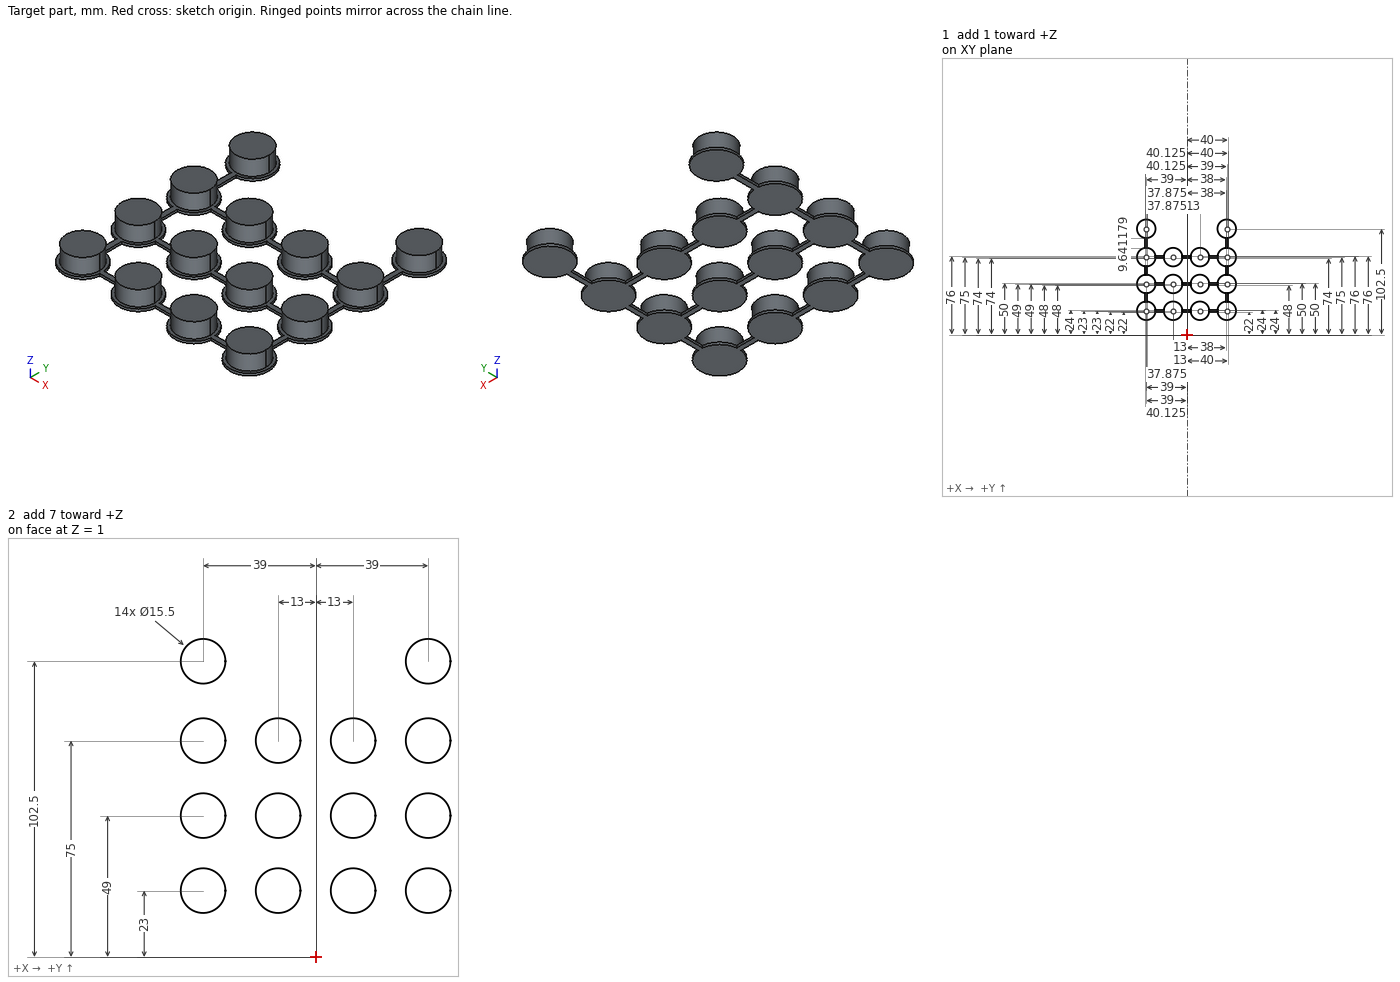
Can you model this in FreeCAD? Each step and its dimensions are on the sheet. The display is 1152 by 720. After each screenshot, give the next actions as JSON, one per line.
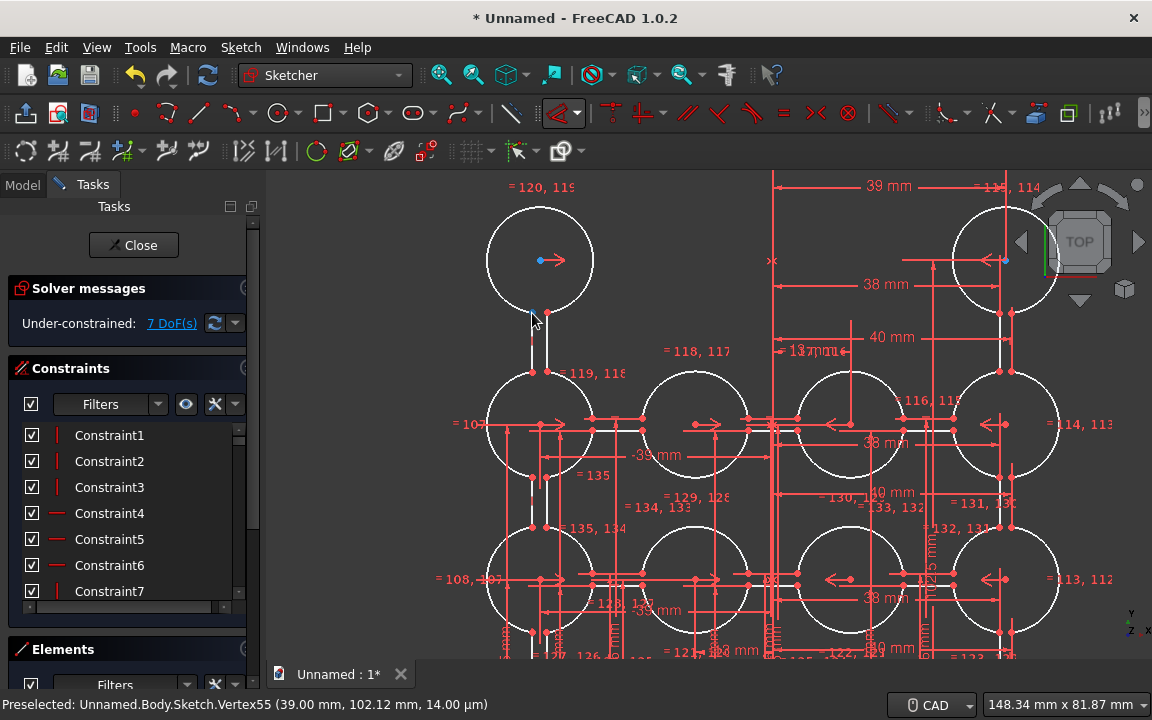
{"action": "left_click", "coordinate": [532, 313]}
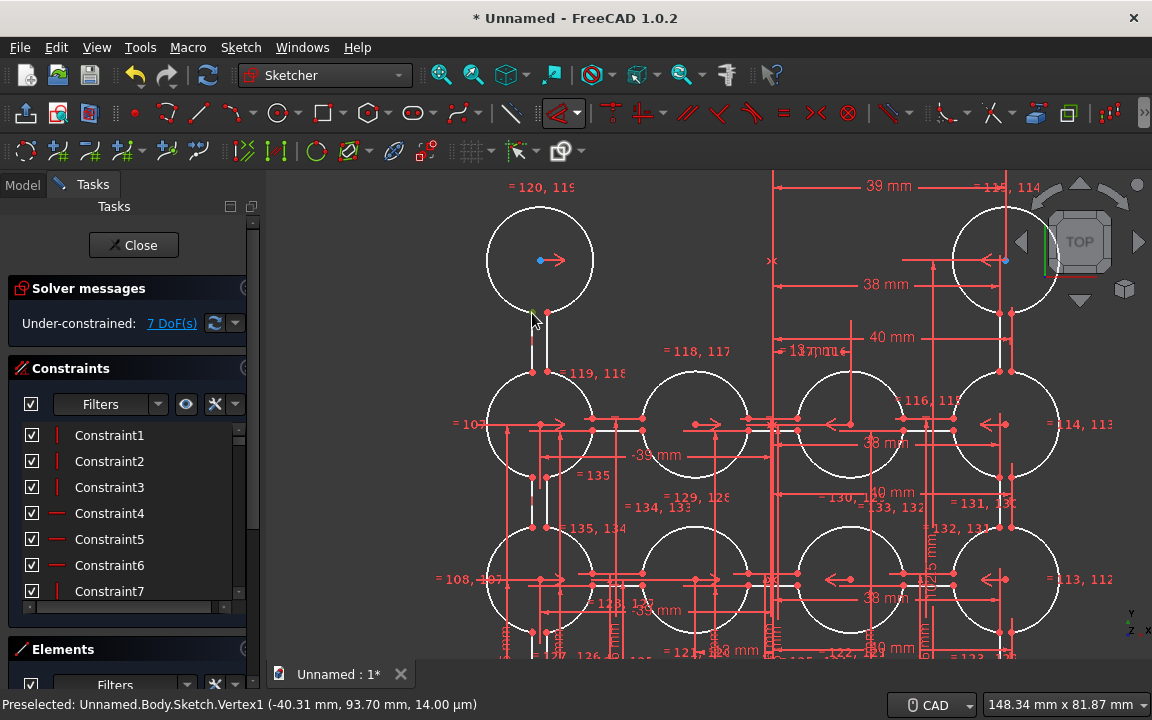
{"action": "key", "text": "l"}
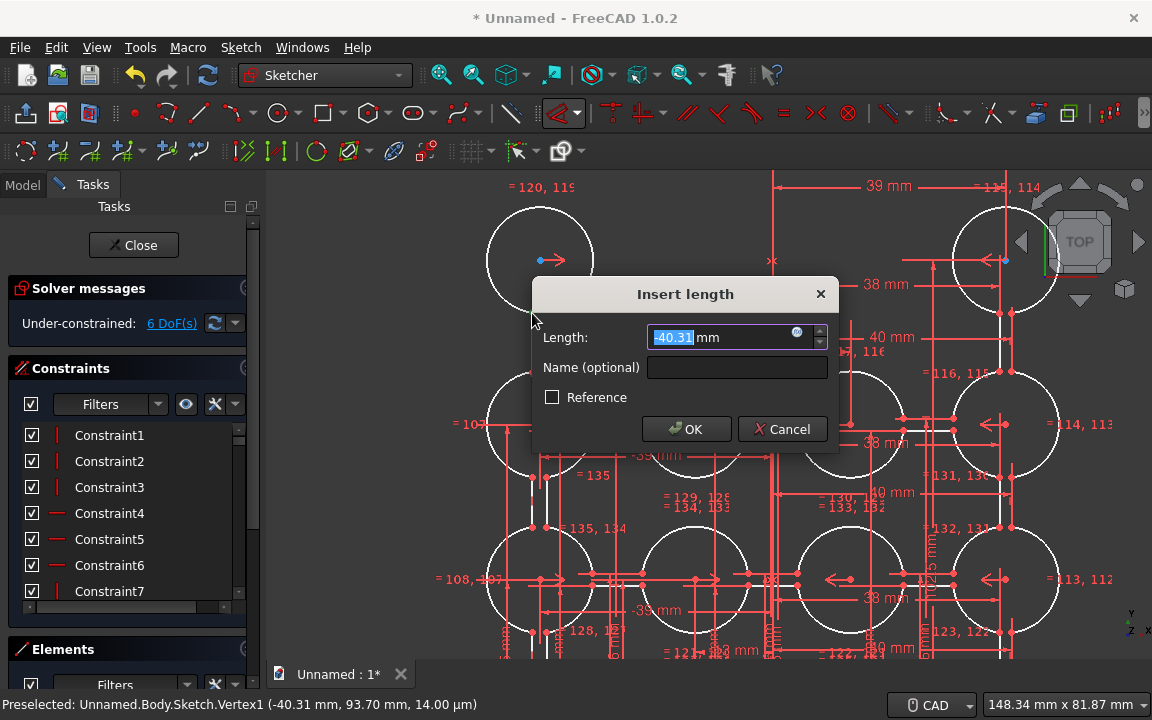
{"action": "type", "text": "-40.125"}
{"action": "key", "text": "Return"}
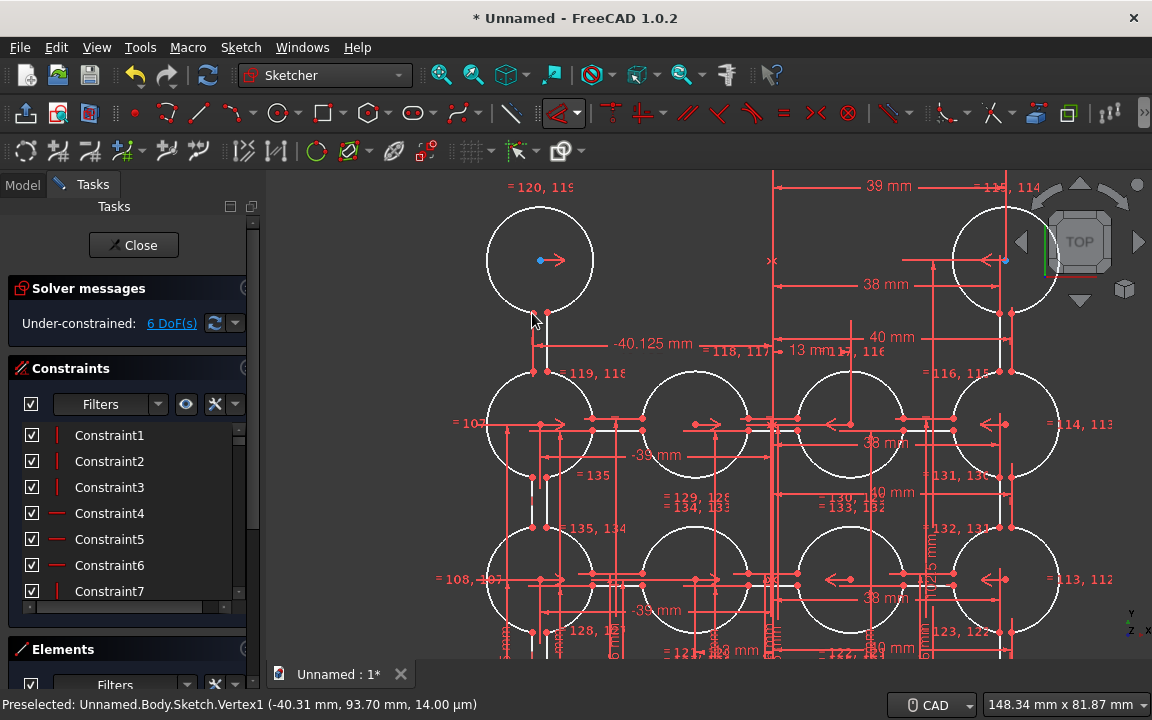
{"action": "left_click", "coordinate": [532, 477]}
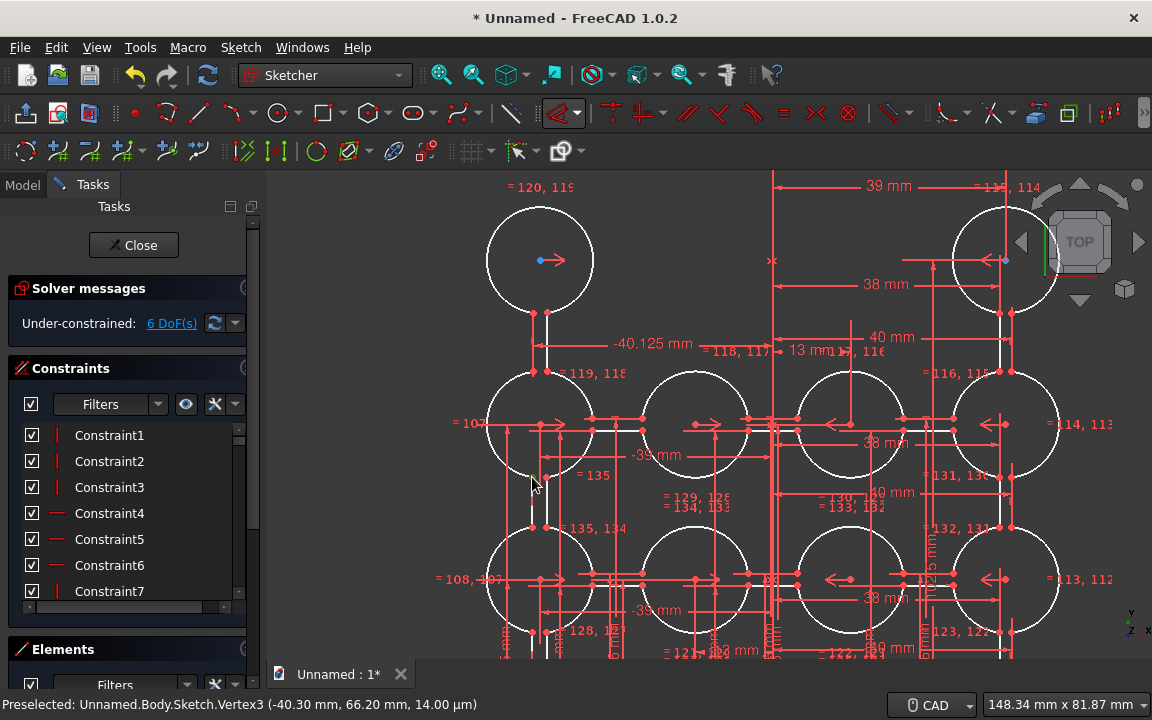
{"action": "left_click", "coordinate": [580, 114]}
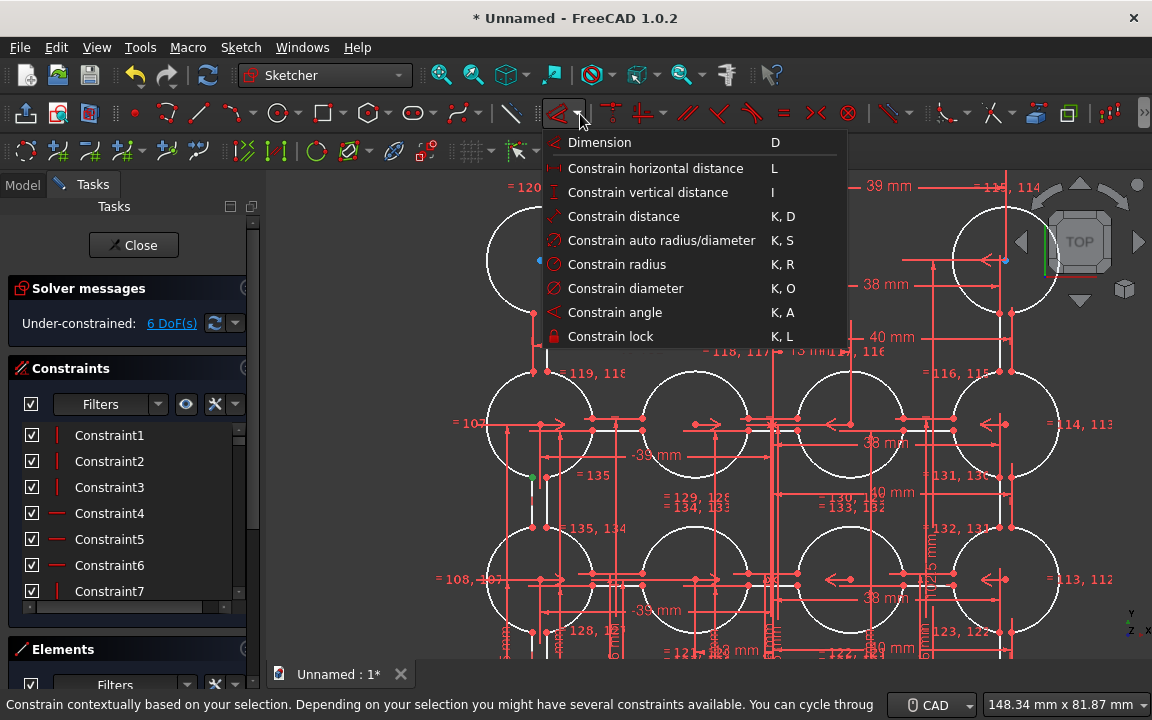
{"action": "left_click", "coordinate": [695, 168]}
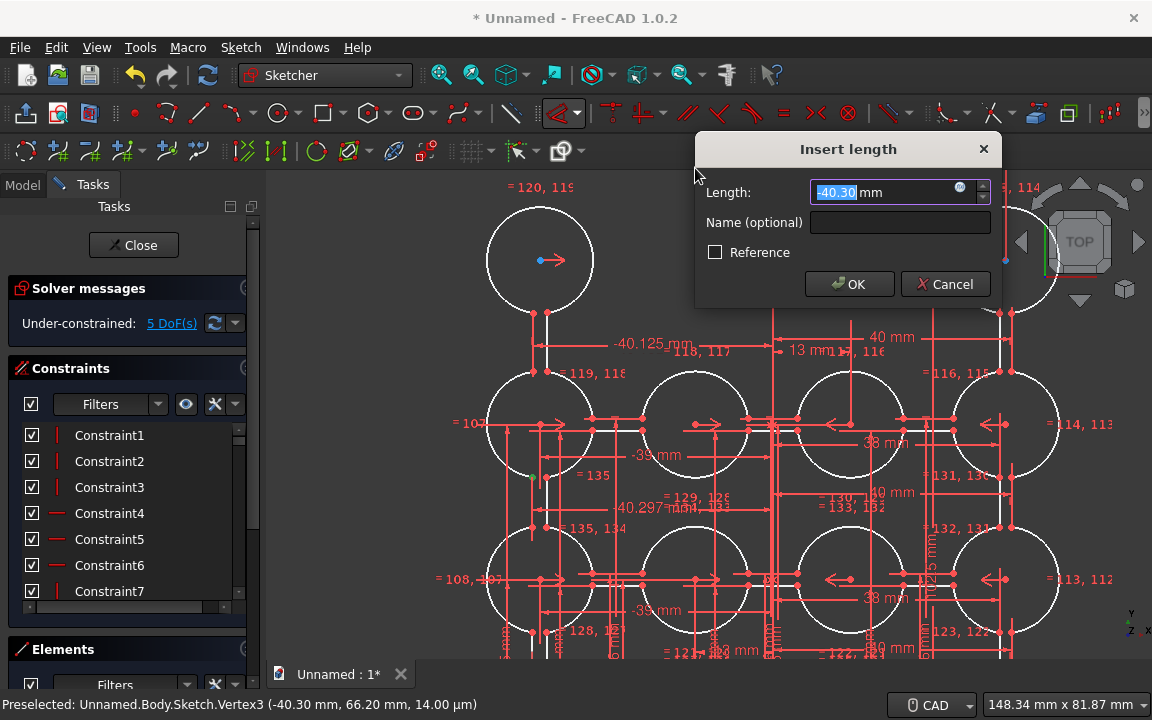
{"action": "type", "text": "-40.125"}
{"action": "key", "text": "Return"}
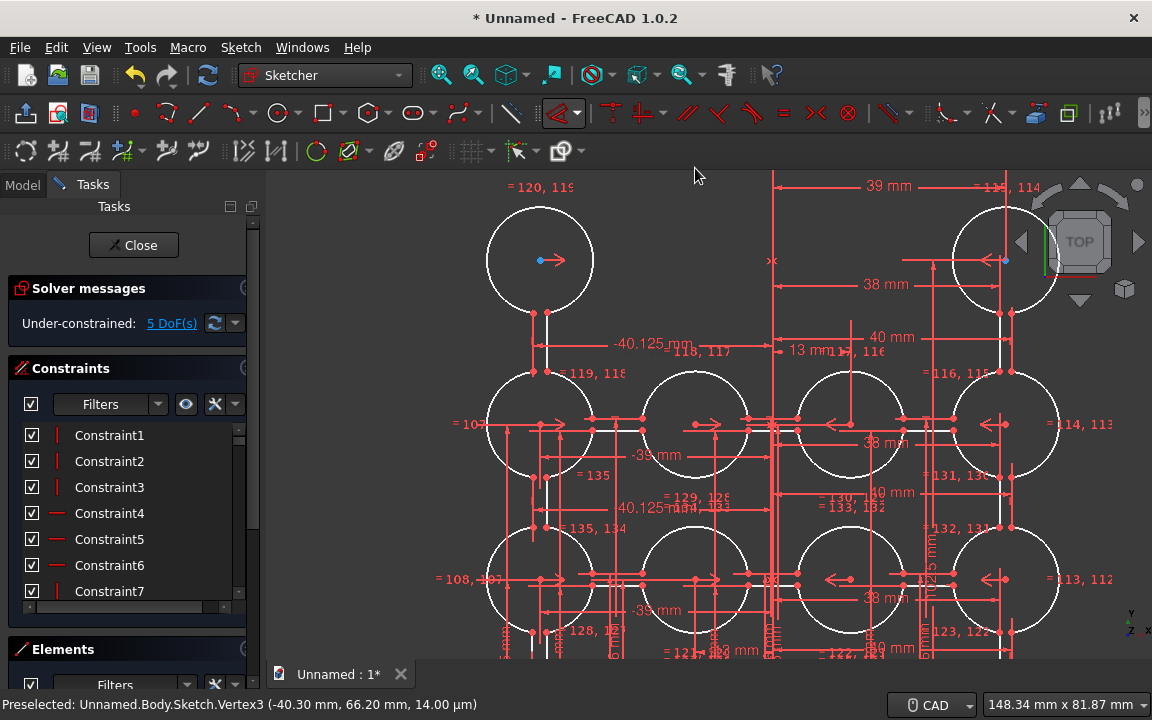
{"action": "scroll", "coordinate": [532, 312], "scroll_direction": "down", "scroll_amount": 4}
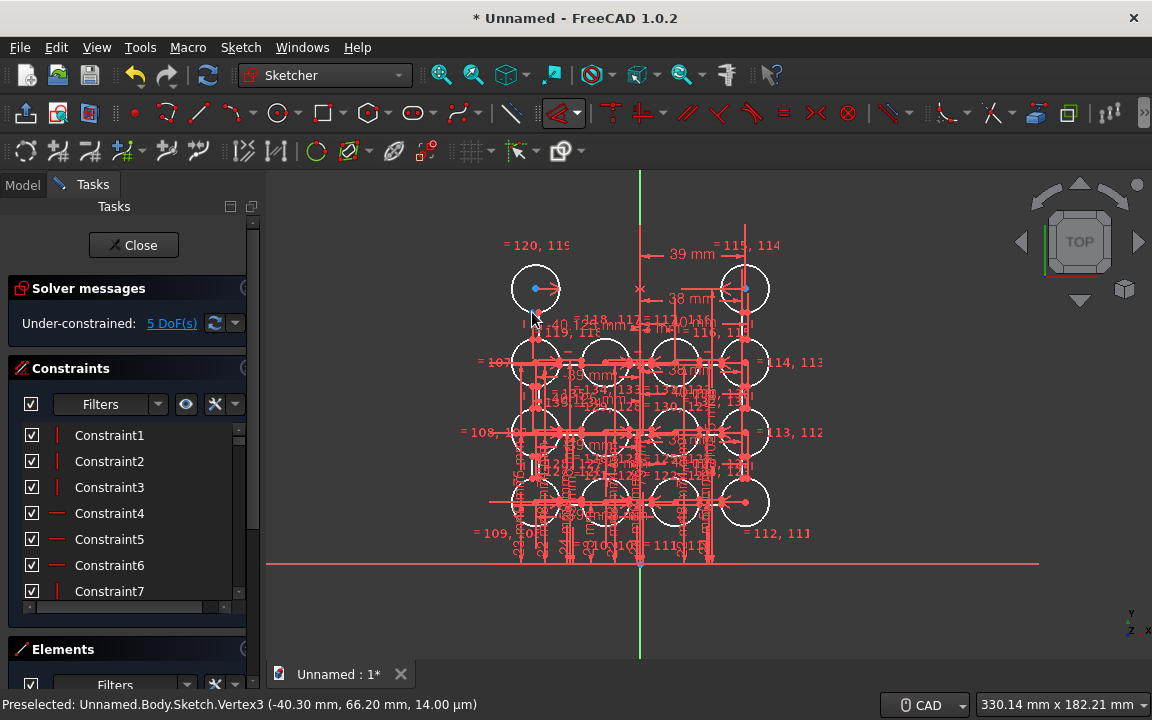
{"action": "scroll", "coordinate": [532, 456], "scroll_direction": "up", "scroll_amount": 4}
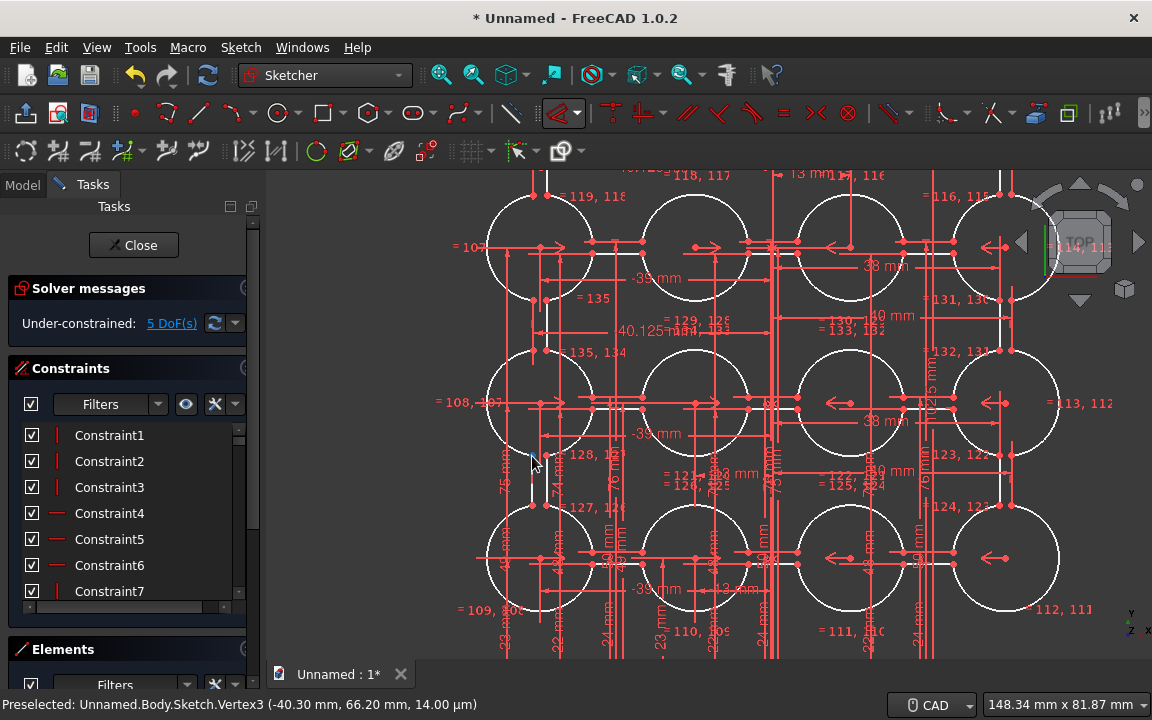
{"action": "left_click", "coordinate": [532, 456]}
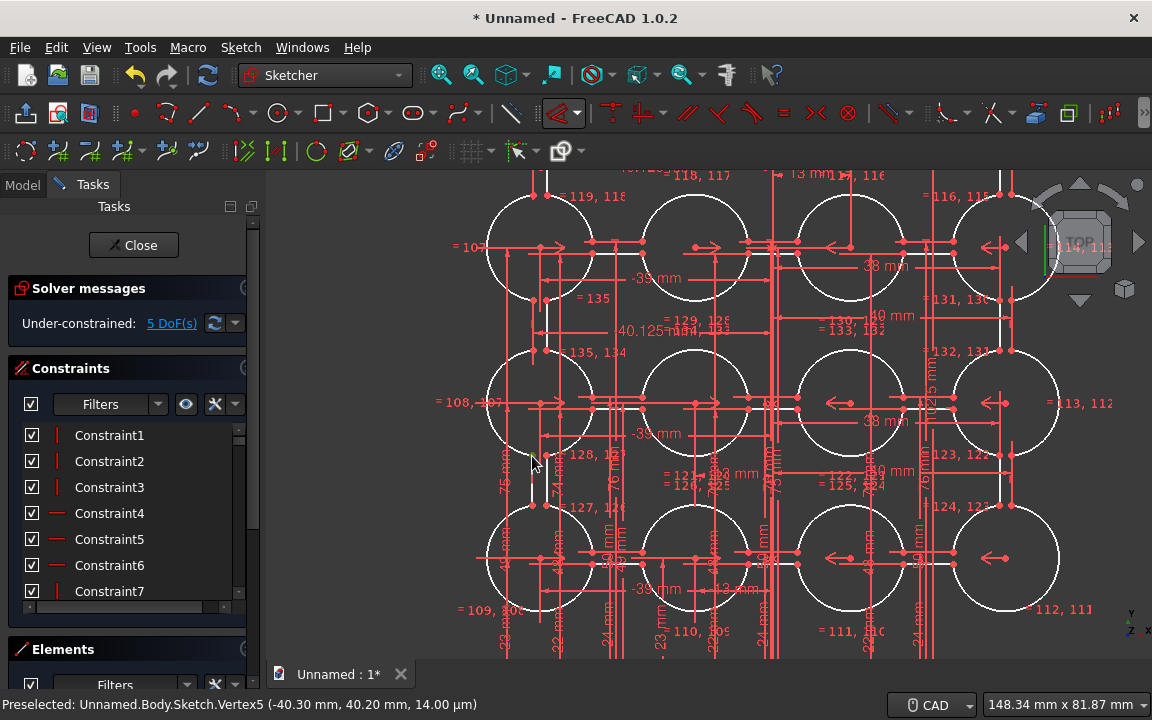
{"action": "key", "text": "l"}